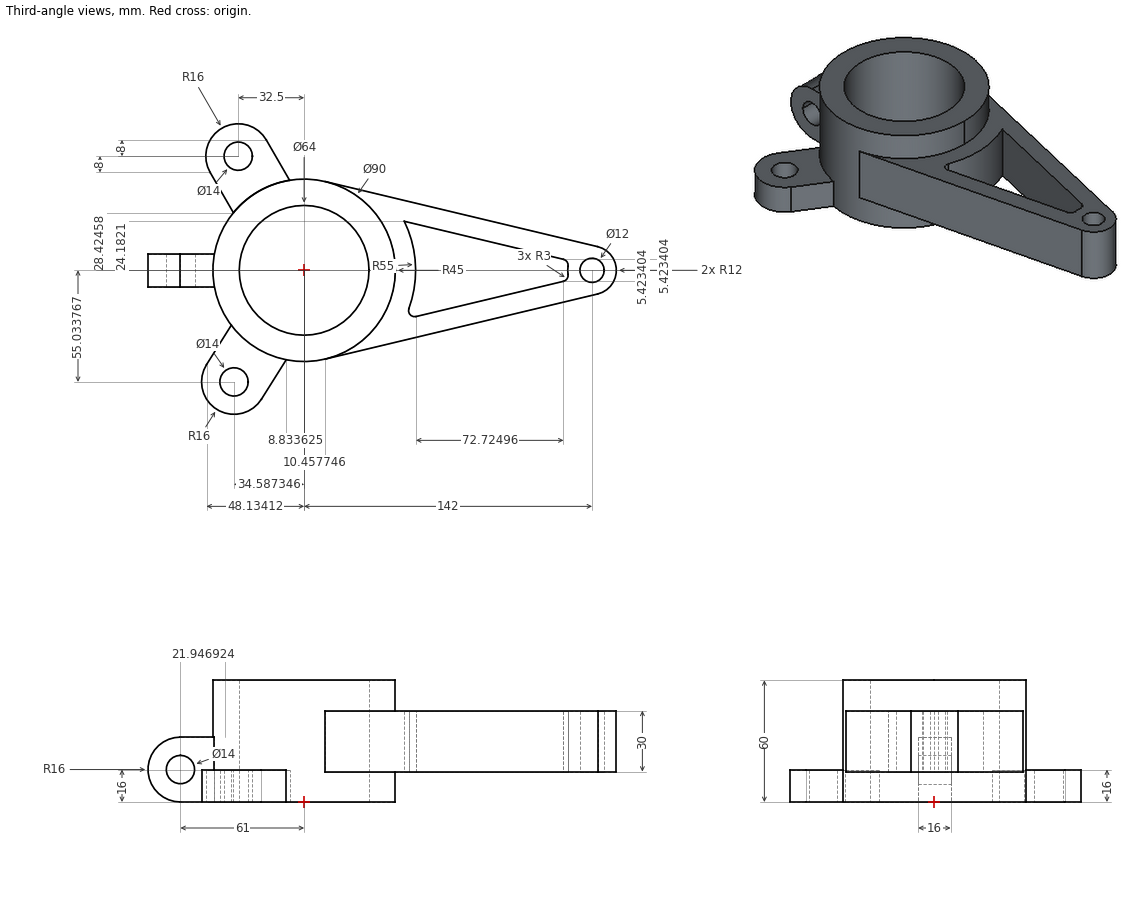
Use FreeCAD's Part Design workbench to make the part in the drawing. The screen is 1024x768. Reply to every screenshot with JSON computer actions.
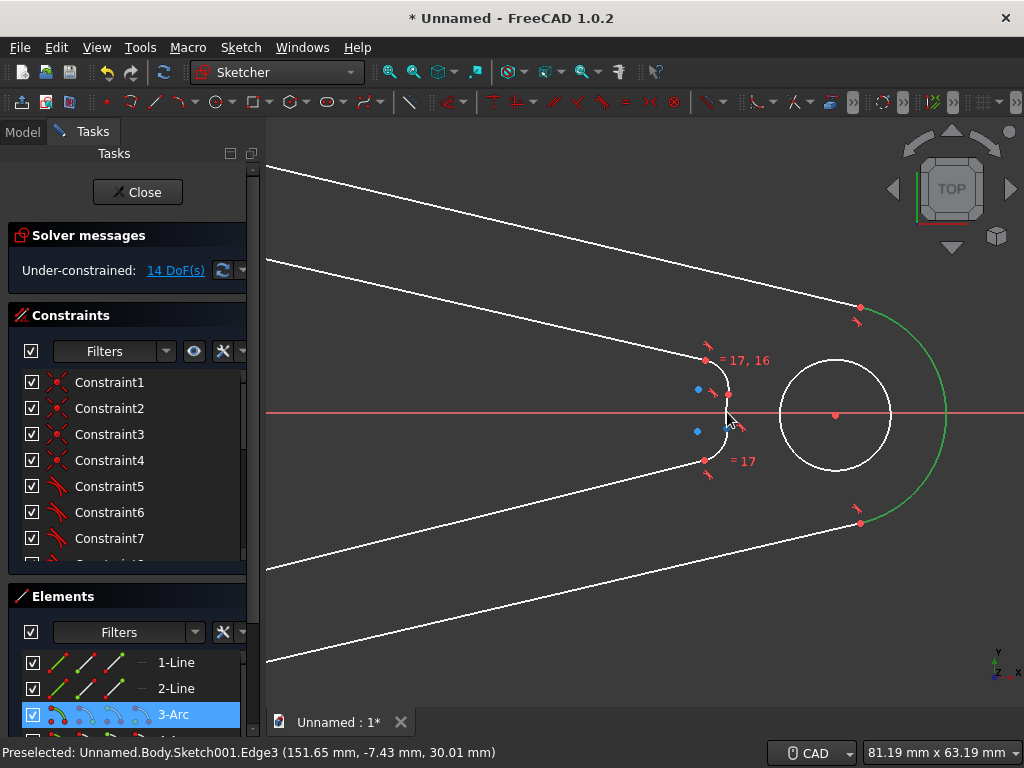
{"action": "left_click", "coordinate": [726, 411]}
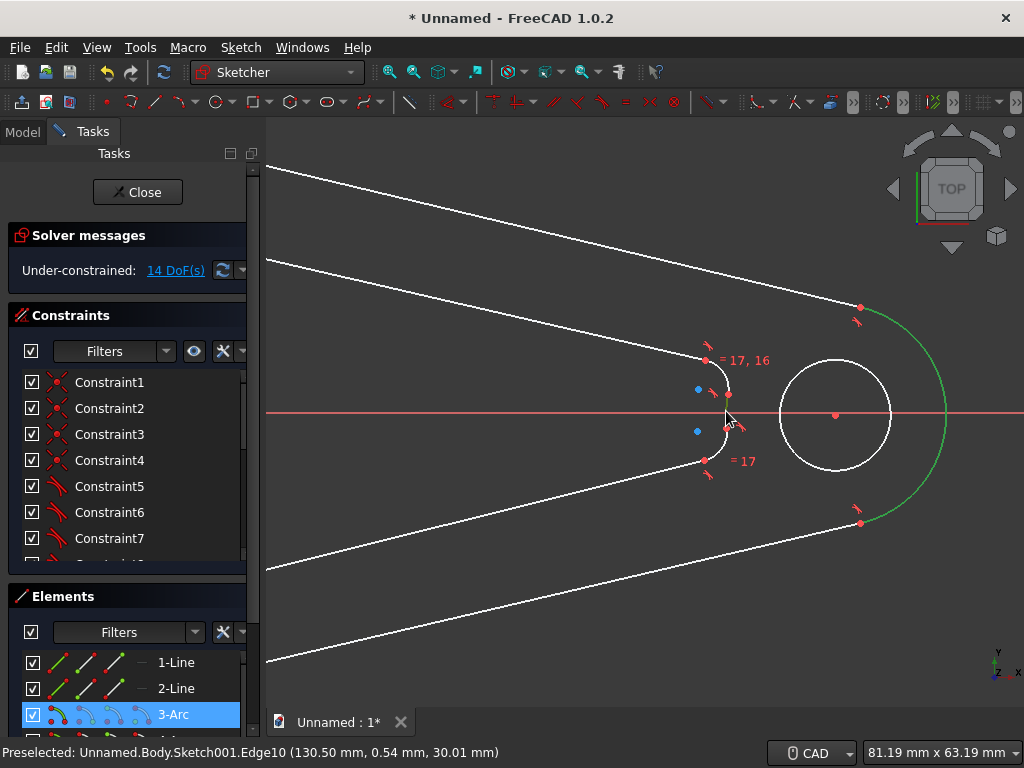
{"action": "left_click", "coordinate": [626, 102]}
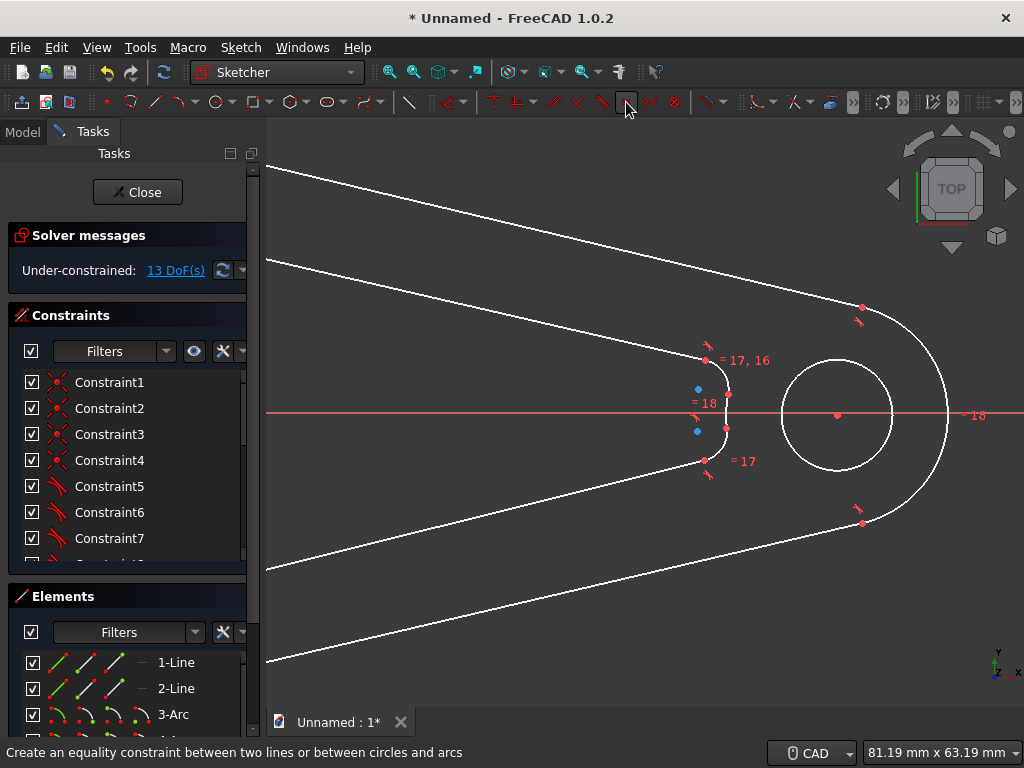
{"action": "left_click", "coordinate": [837, 415]}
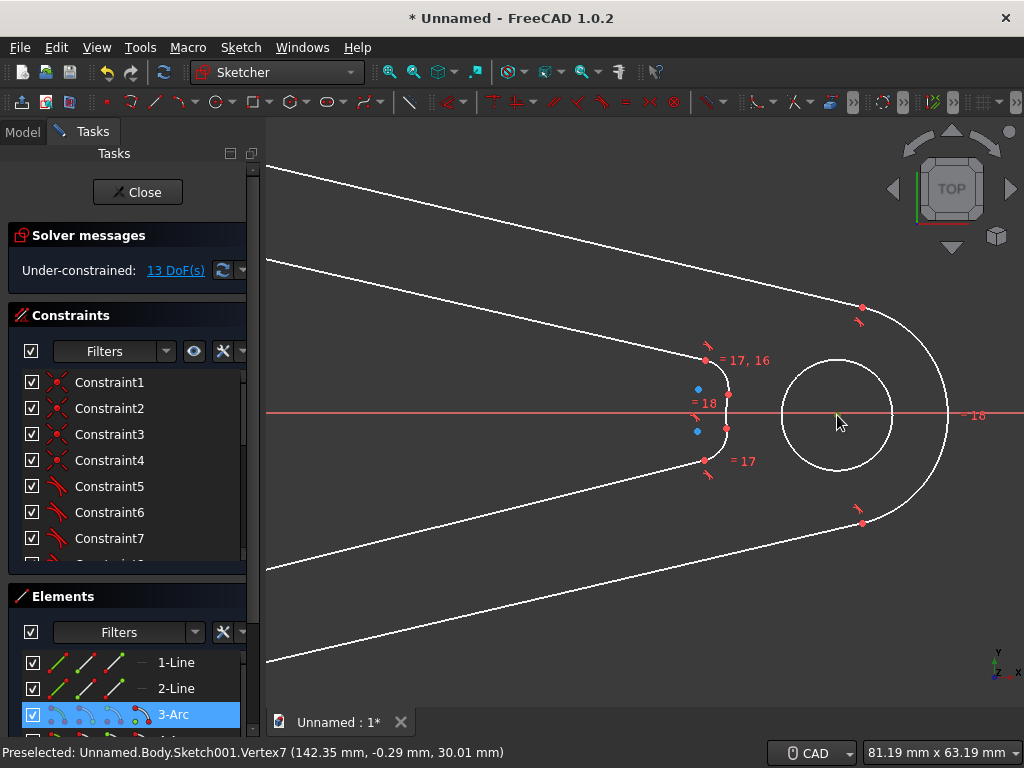
{"action": "left_click", "coordinate": [334, 413]}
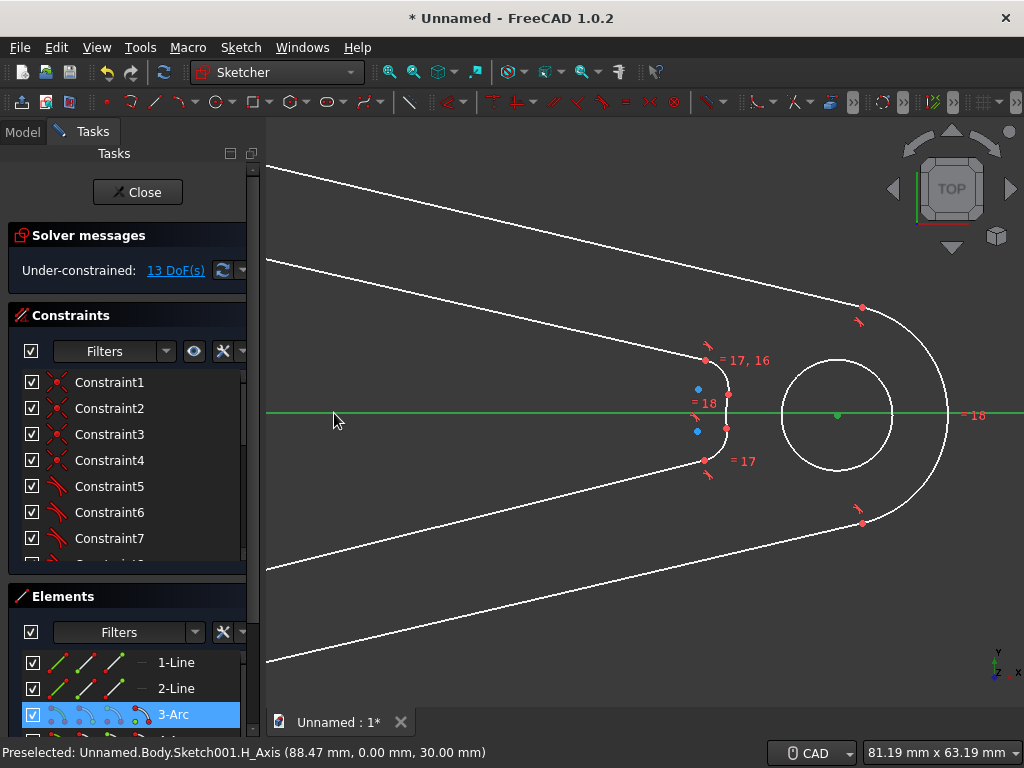
{"action": "key", "text": "c"}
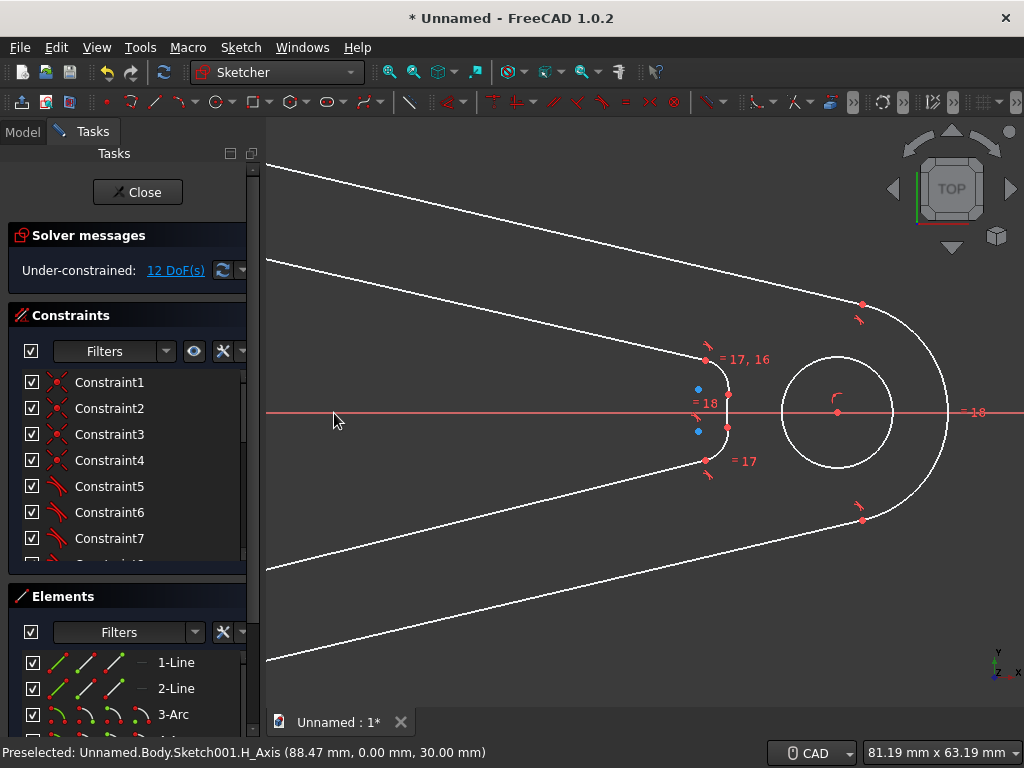
{"action": "key", "text": "d"}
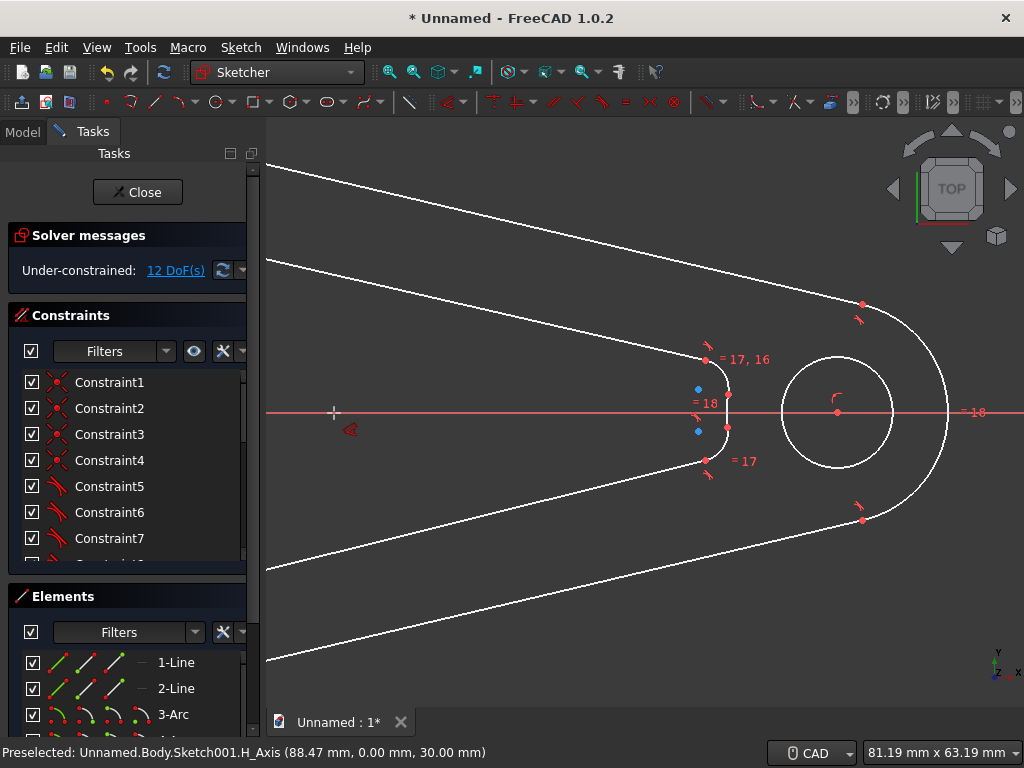
{"action": "scroll", "coordinate": [727, 412], "scroll_direction": "down", "scroll_amount": 6}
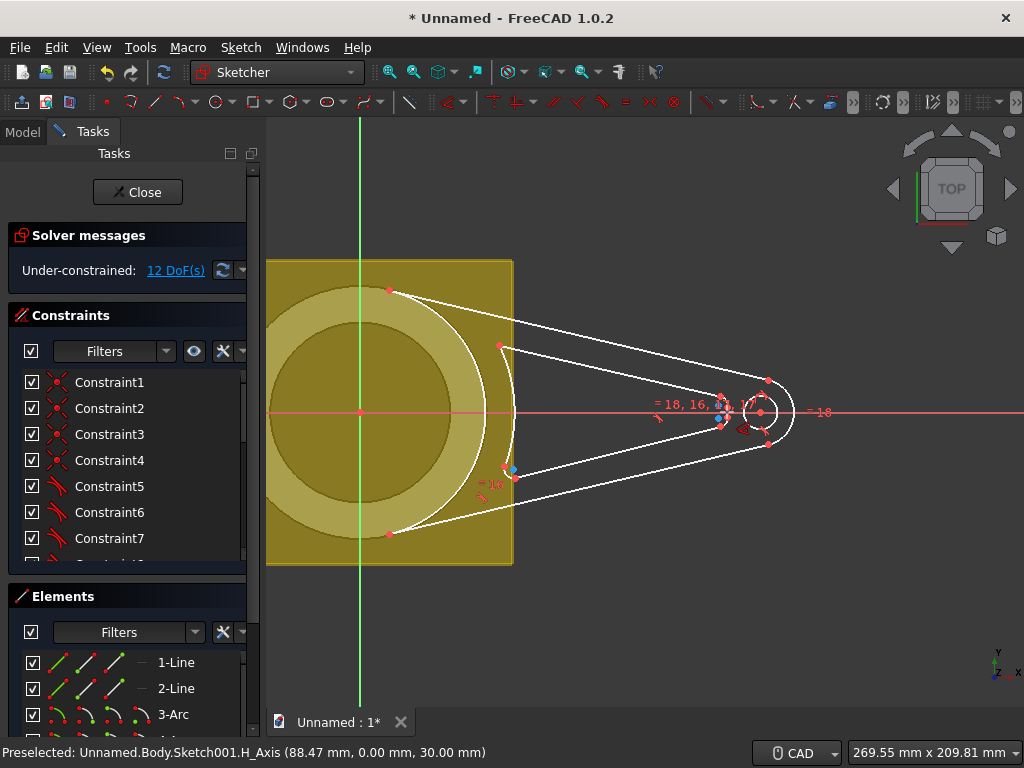
{"action": "left_click", "coordinate": [789, 430]}
{"action": "left_click", "coordinate": [816, 447]}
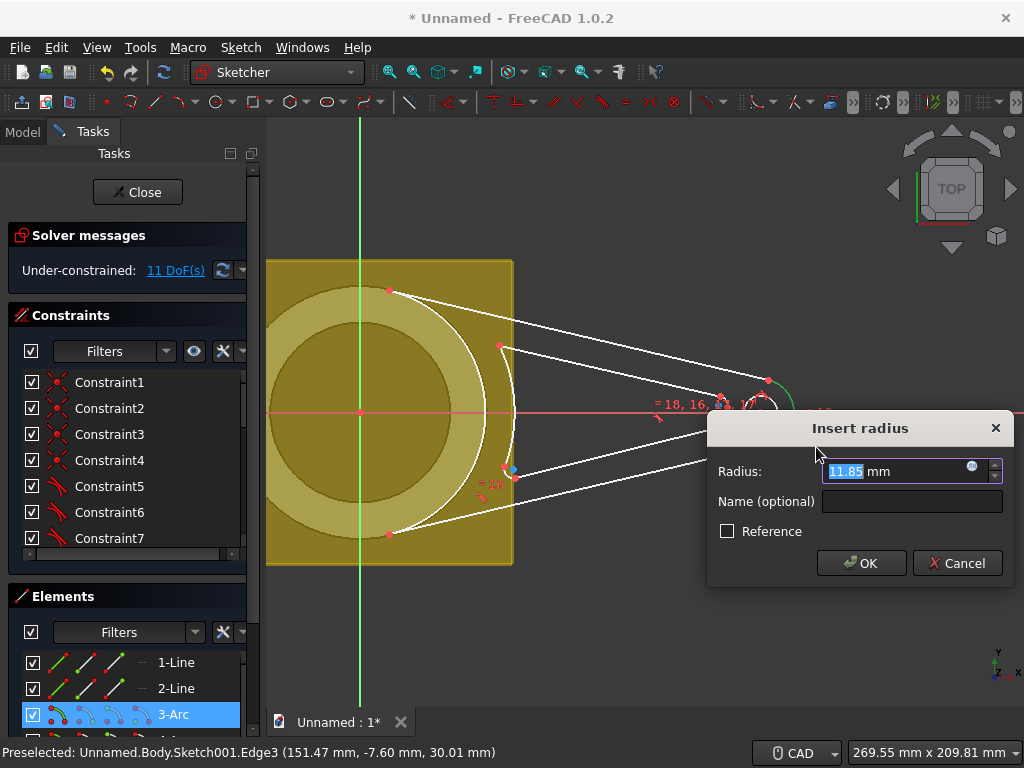
{"action": "type", "text": "12"}
{"action": "key", "text": "Return"}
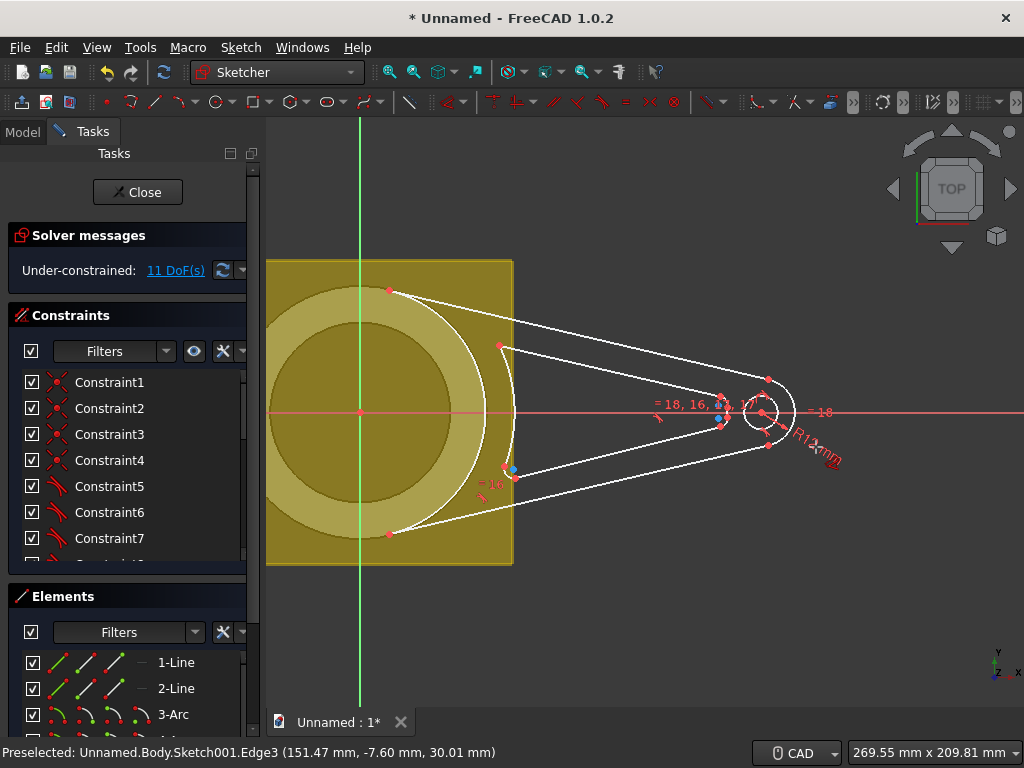
{"action": "left_click", "coordinate": [468, 476]}
{"action": "left_click", "coordinate": [496, 492]}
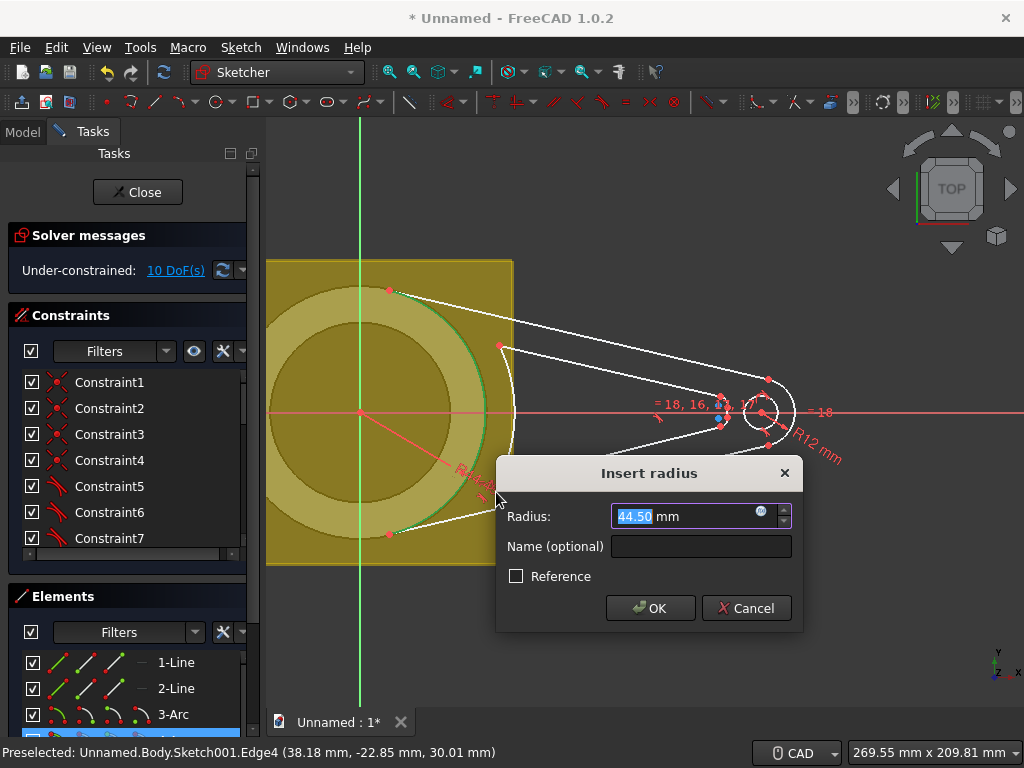
{"action": "type", "text": "45"}
{"action": "key", "text": "Return"}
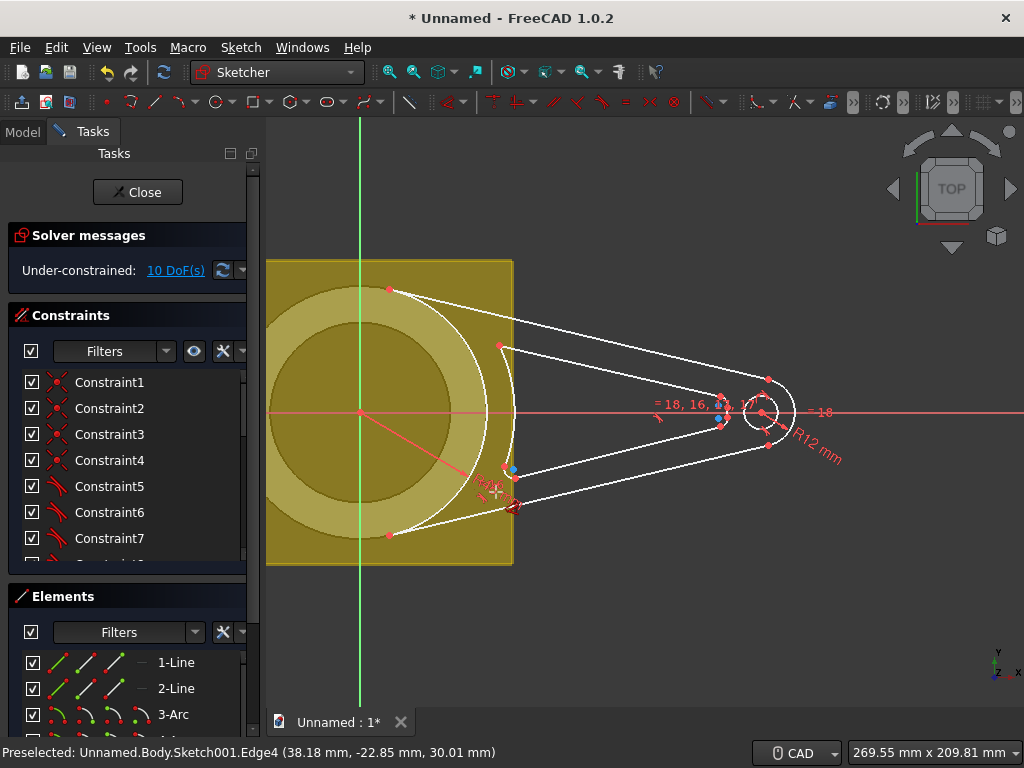
{"action": "scroll", "coordinate": [507, 475], "scroll_direction": "up", "scroll_amount": 8}